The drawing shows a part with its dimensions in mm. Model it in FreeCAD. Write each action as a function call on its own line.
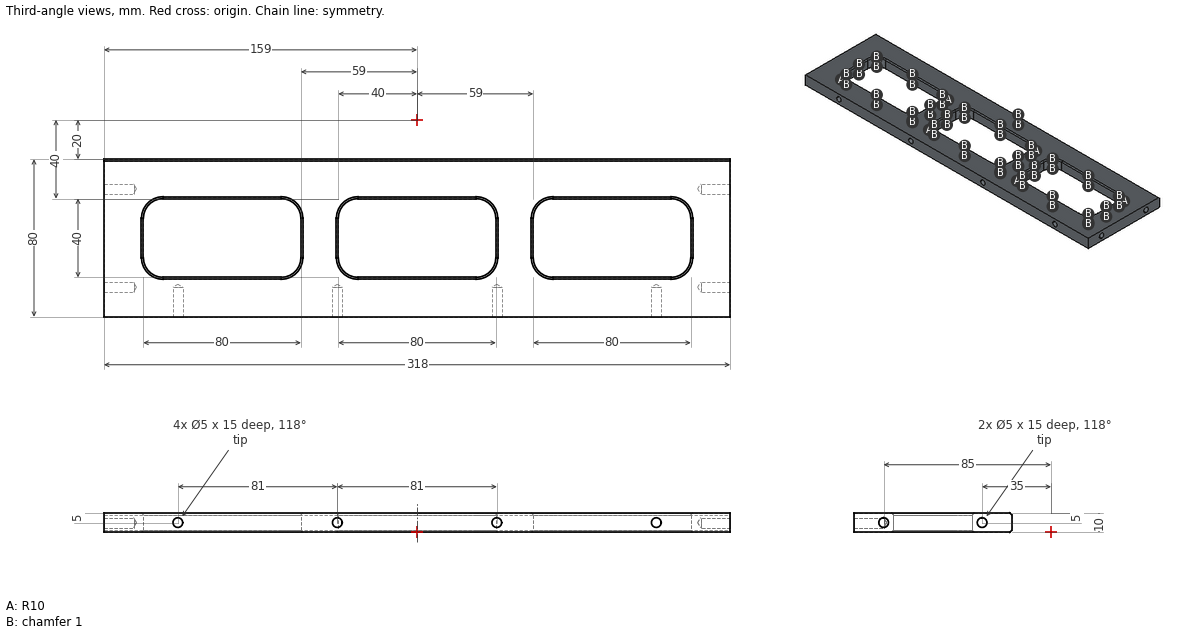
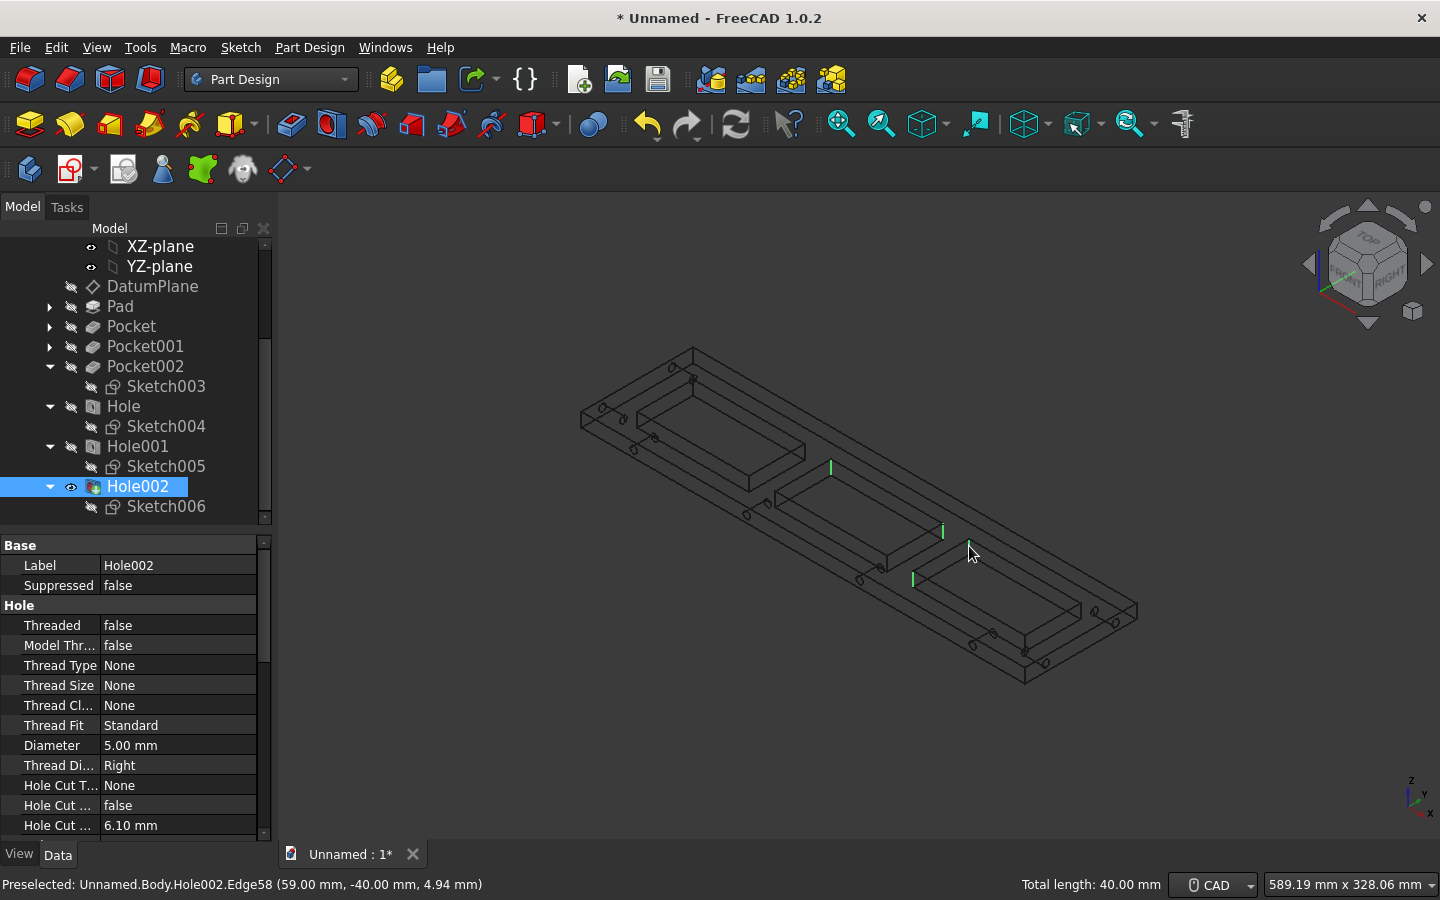
click(1081, 610, ctrl)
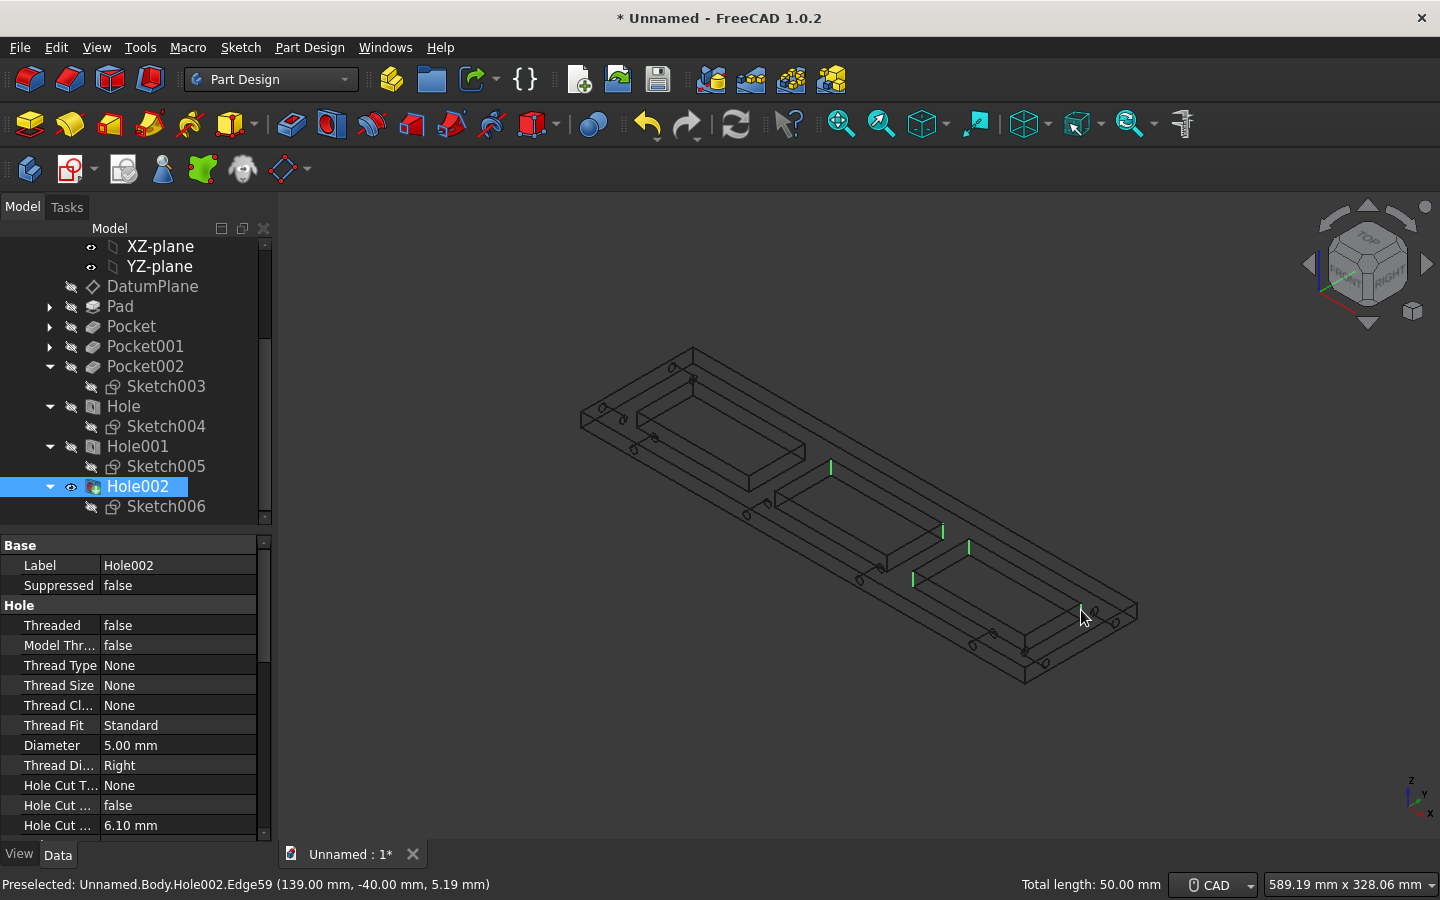
click(805, 451, ctrl)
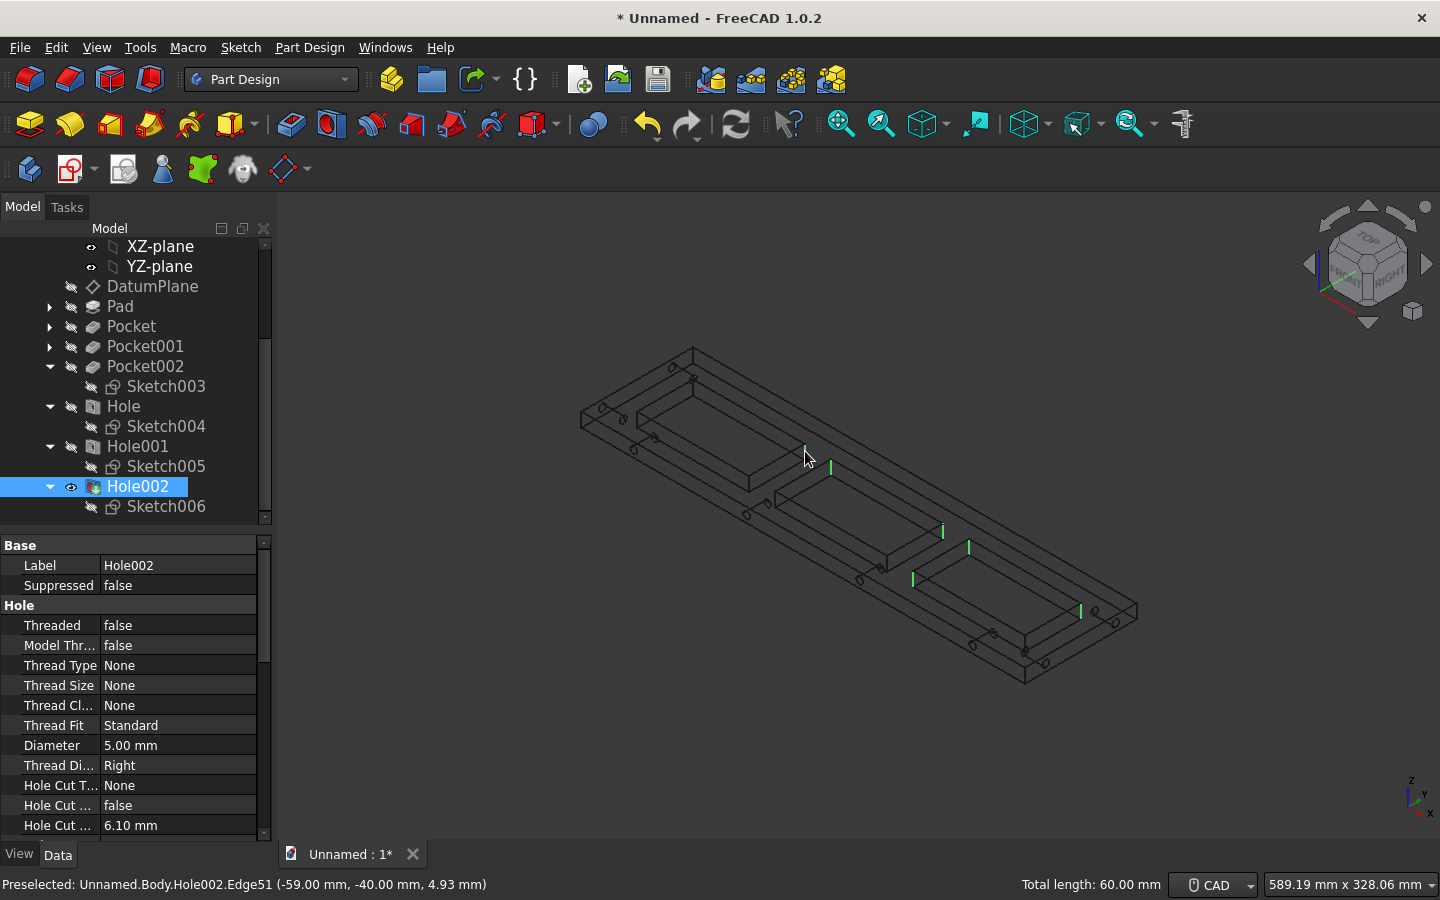
click(693, 386, ctrl)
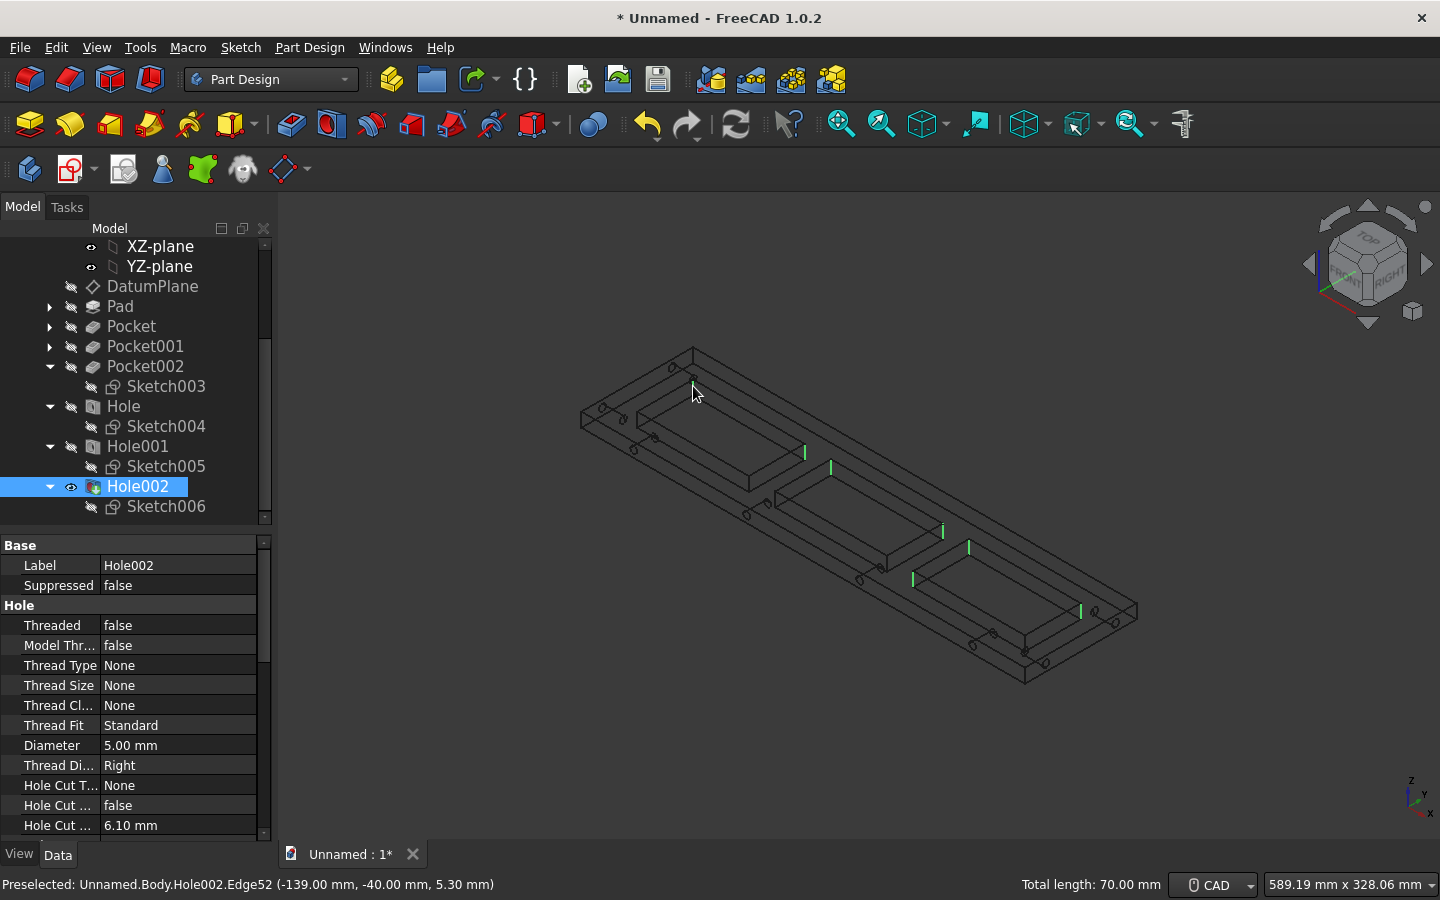
click(637, 419, ctrl)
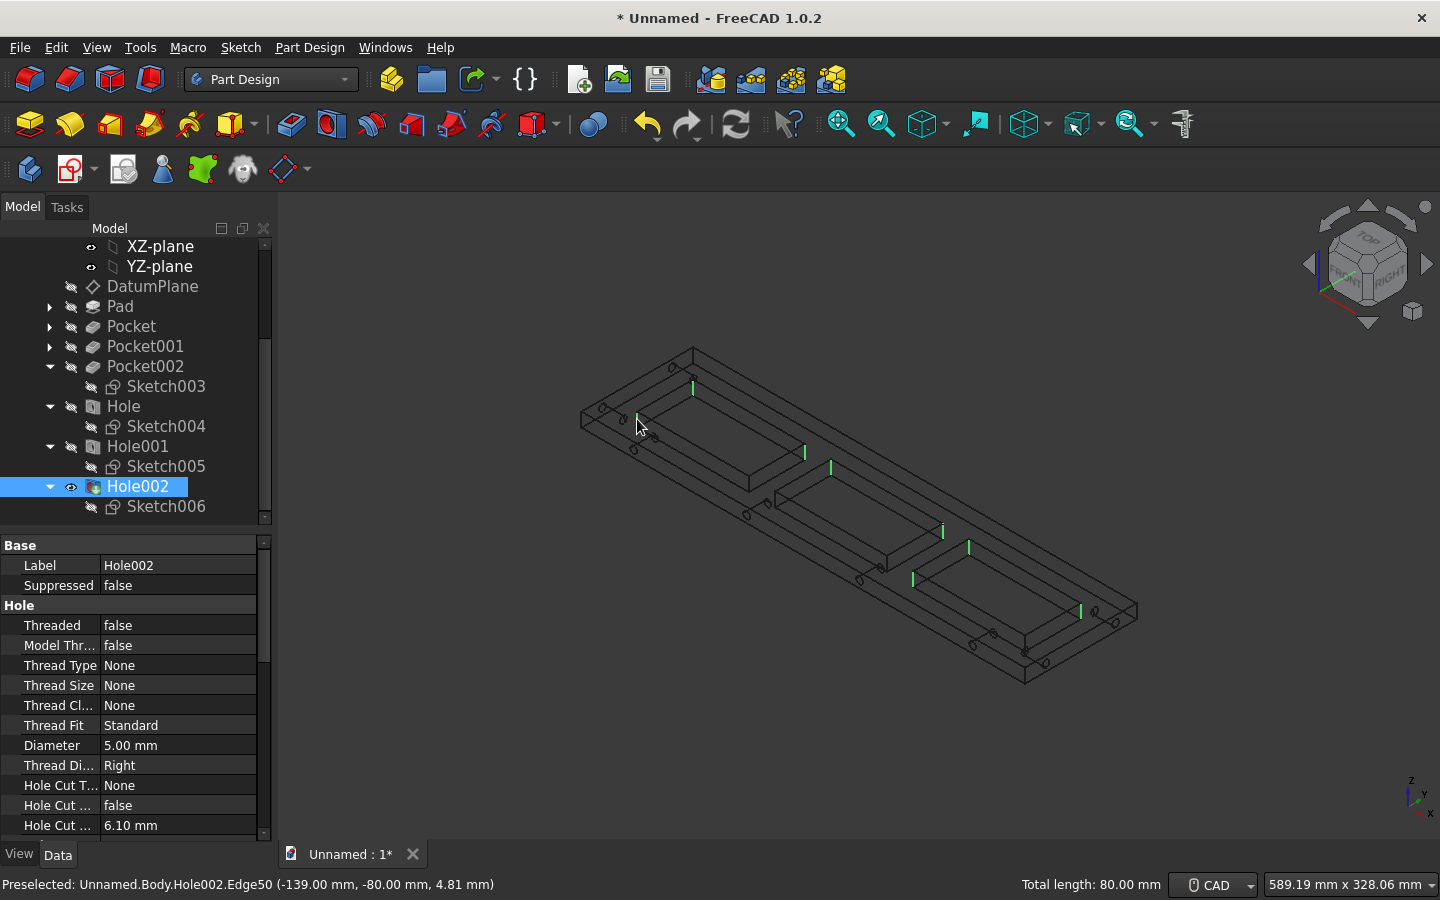
click(749, 483, ctrl)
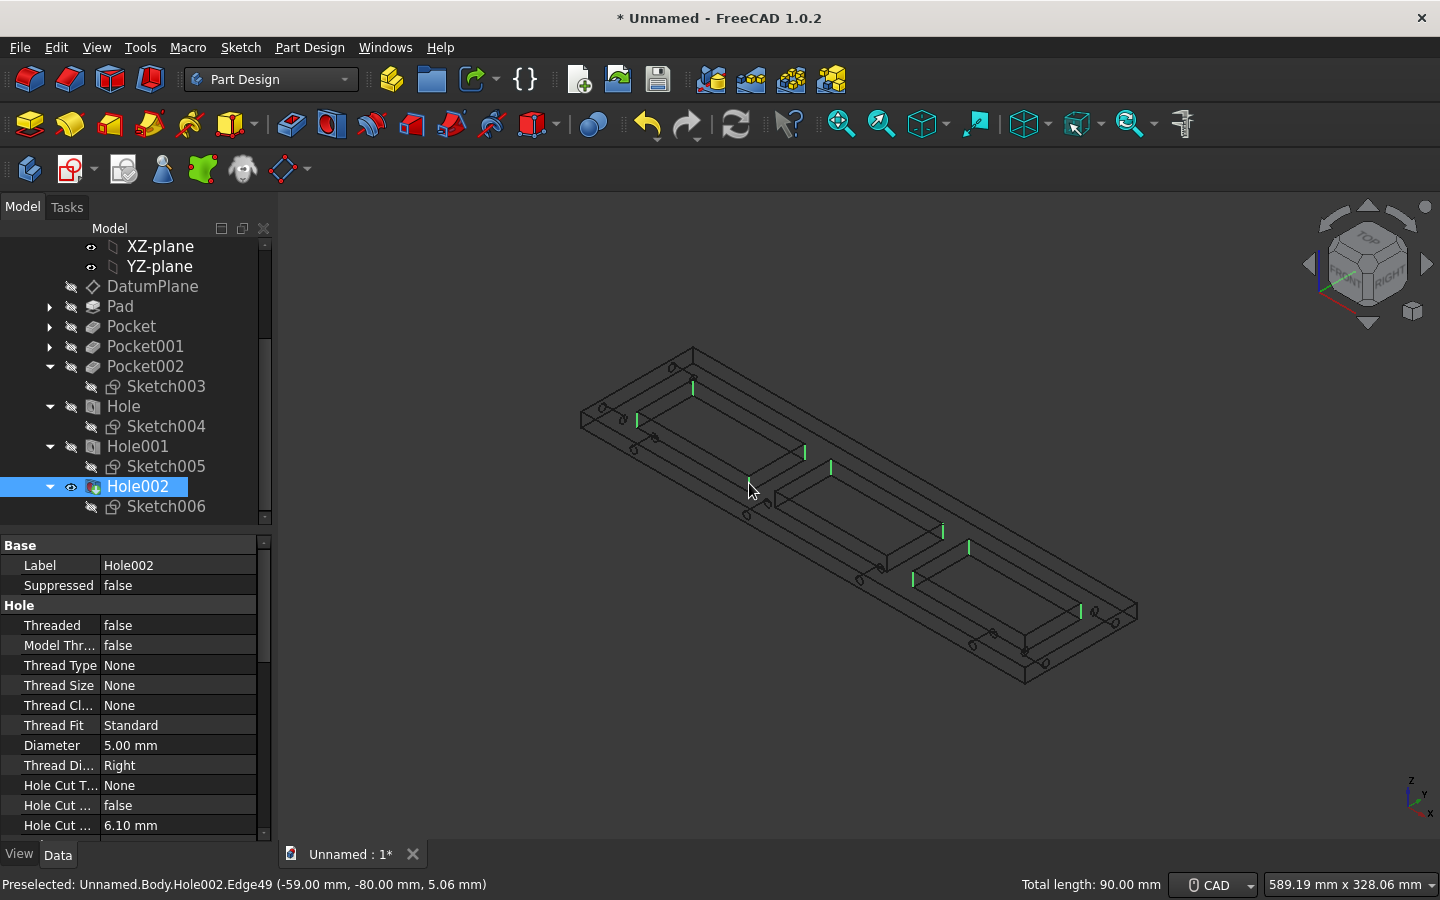
scroll(887, 563, up, 4)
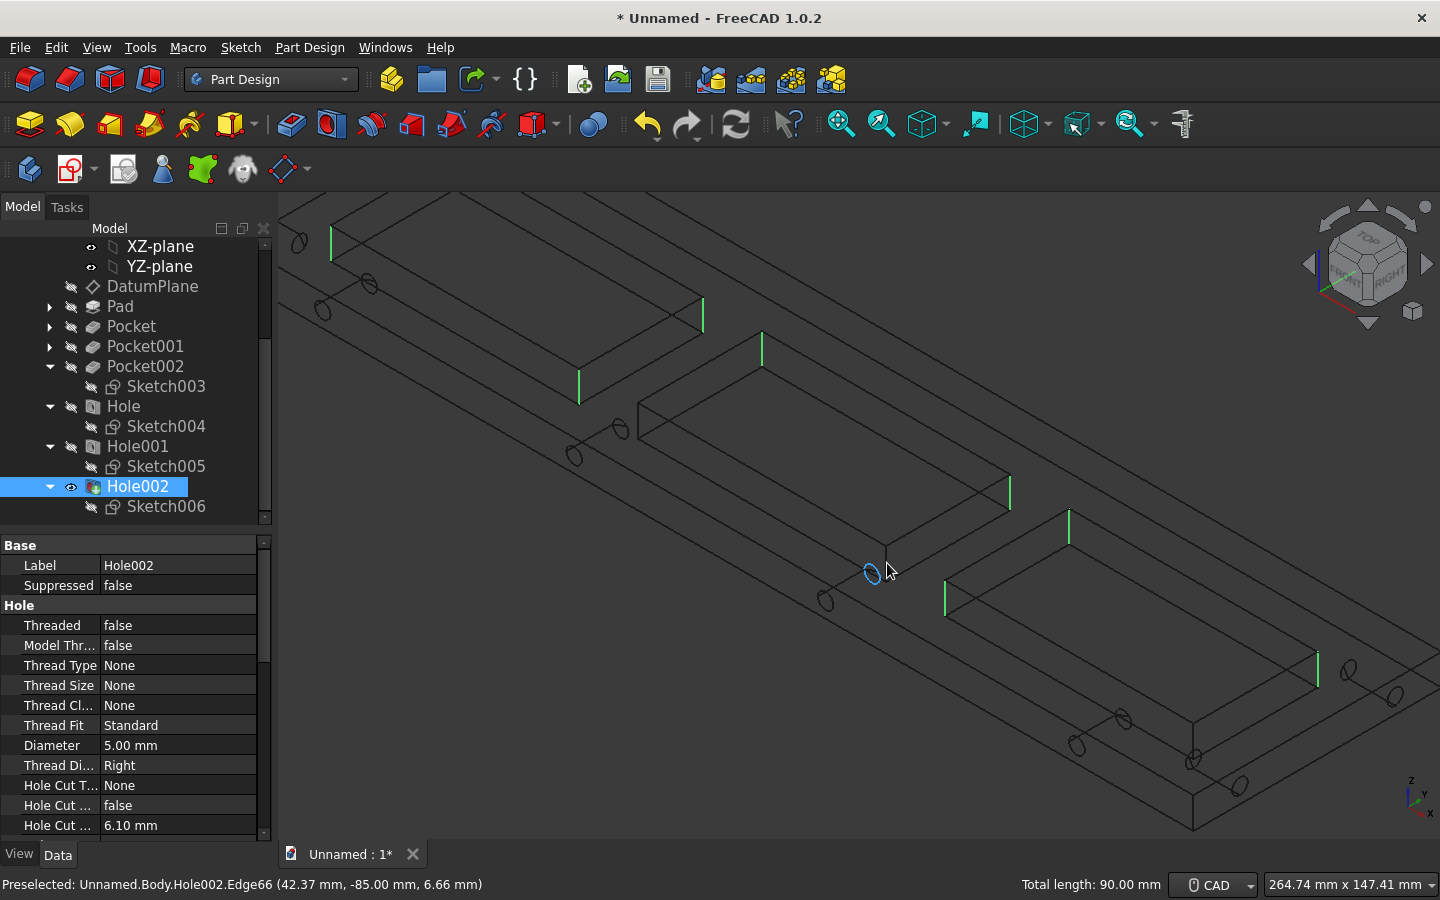
click(886, 563, ctrl)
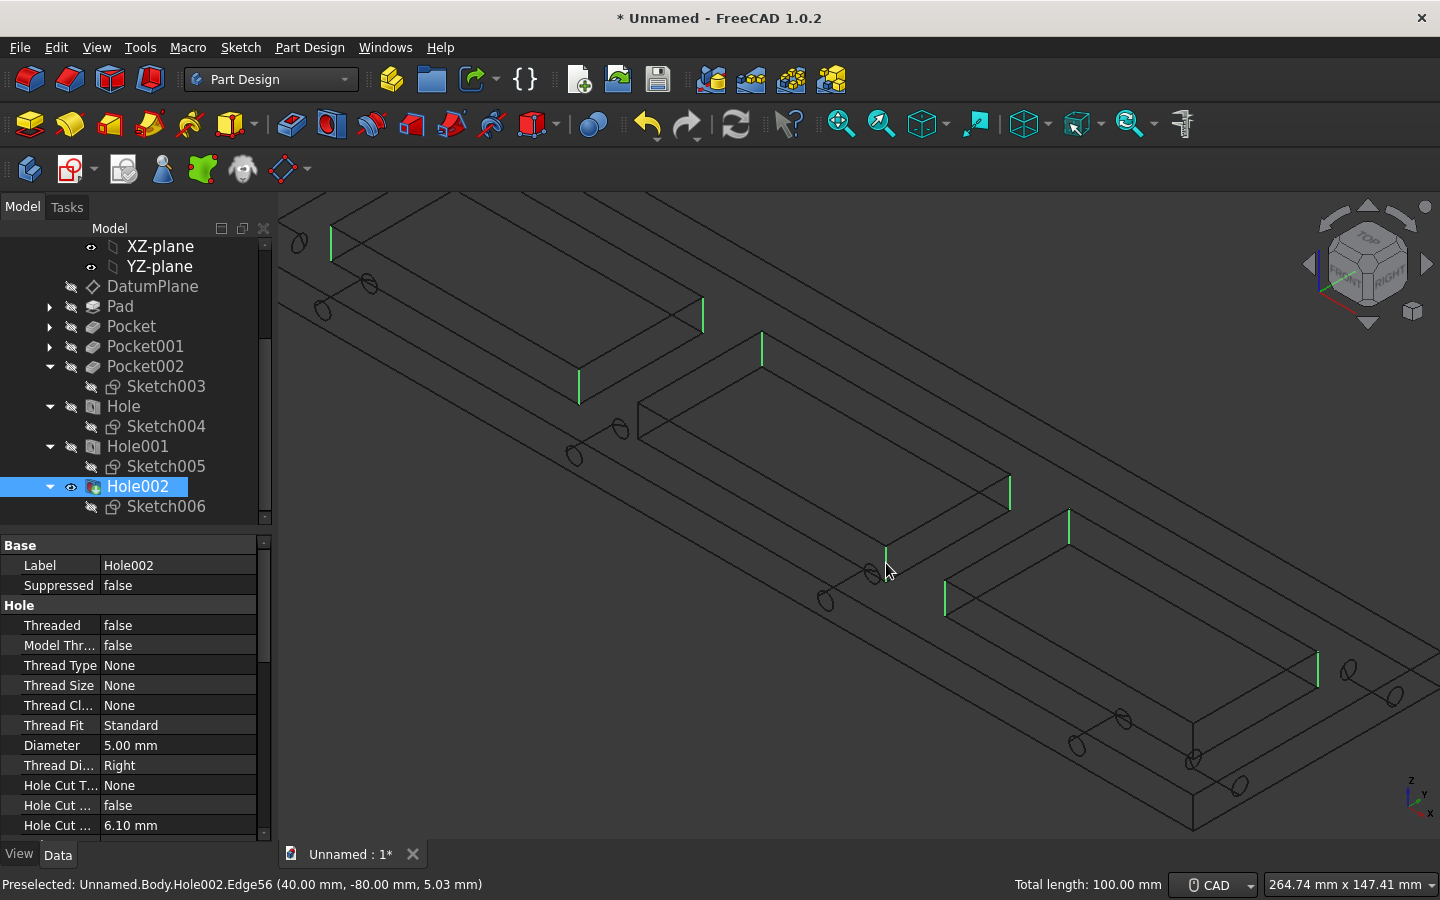
click(638, 420, ctrl)